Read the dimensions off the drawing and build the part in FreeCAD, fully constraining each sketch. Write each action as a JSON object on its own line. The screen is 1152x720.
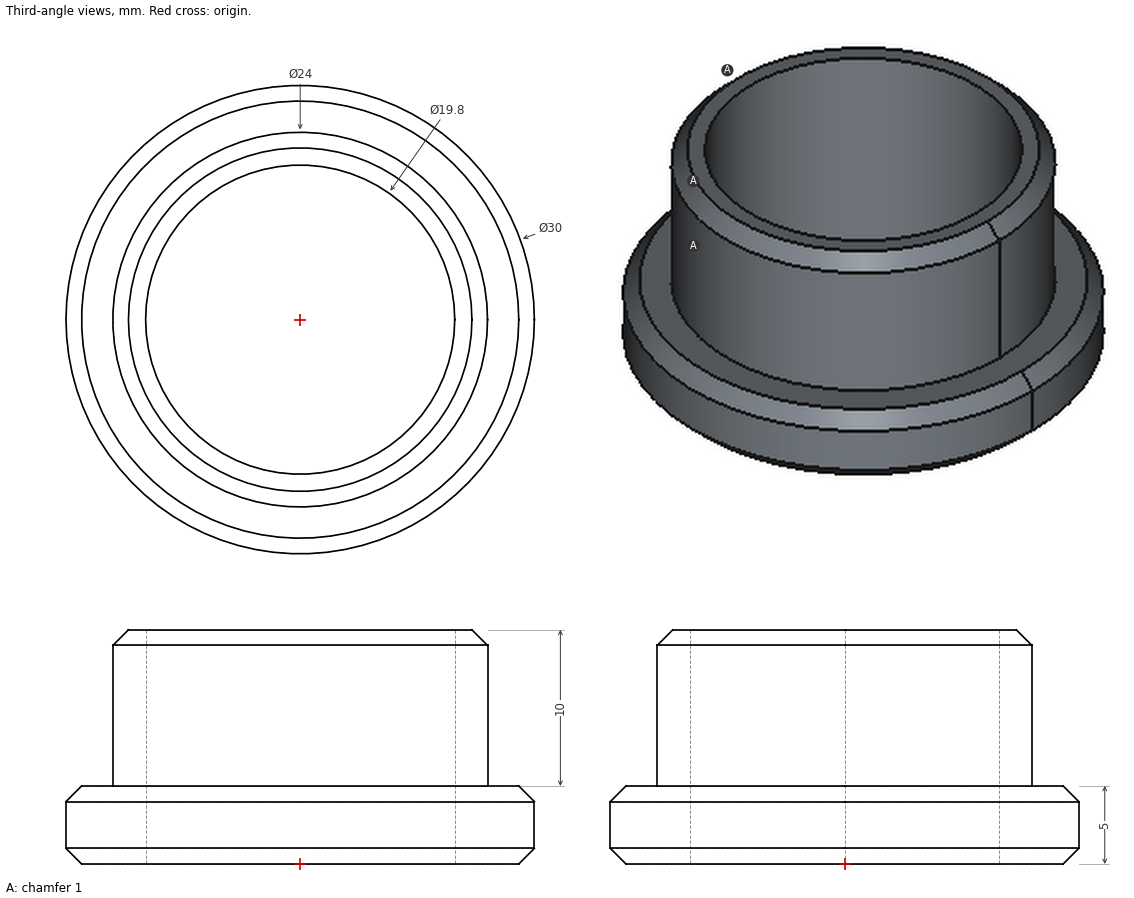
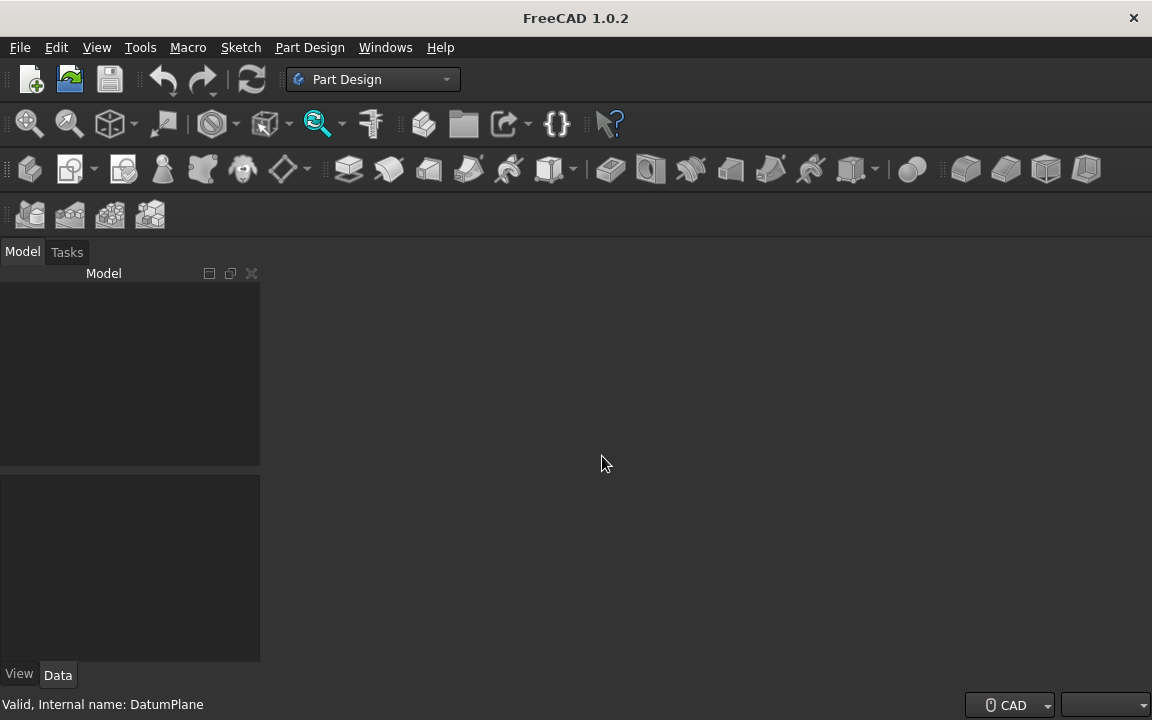
{"action": "left_click", "coordinate": [30, 80]}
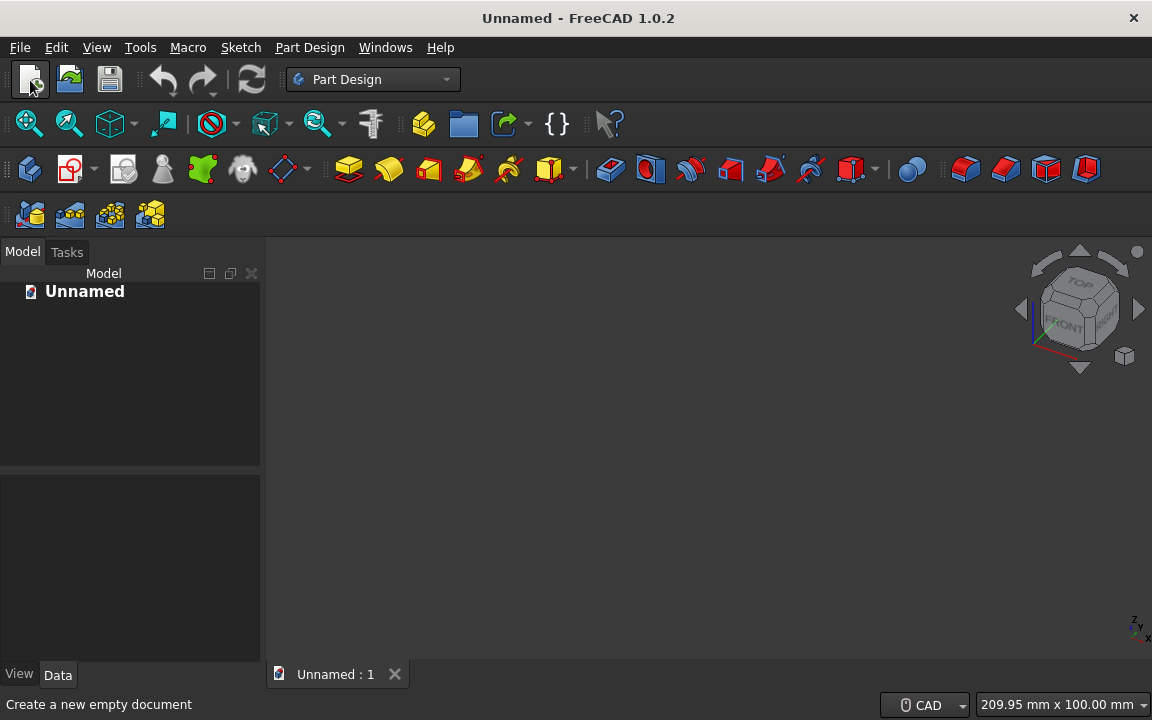
{"action": "left_click", "coordinate": [70, 170]}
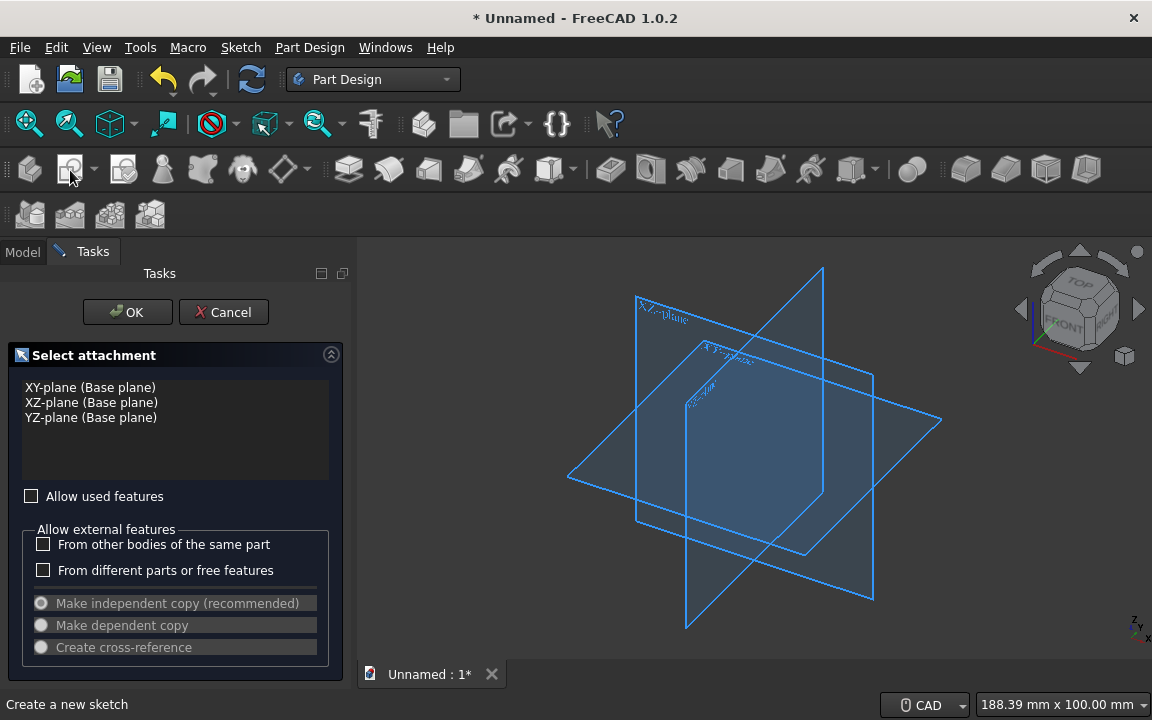
{"action": "left_click", "coordinate": [82, 388]}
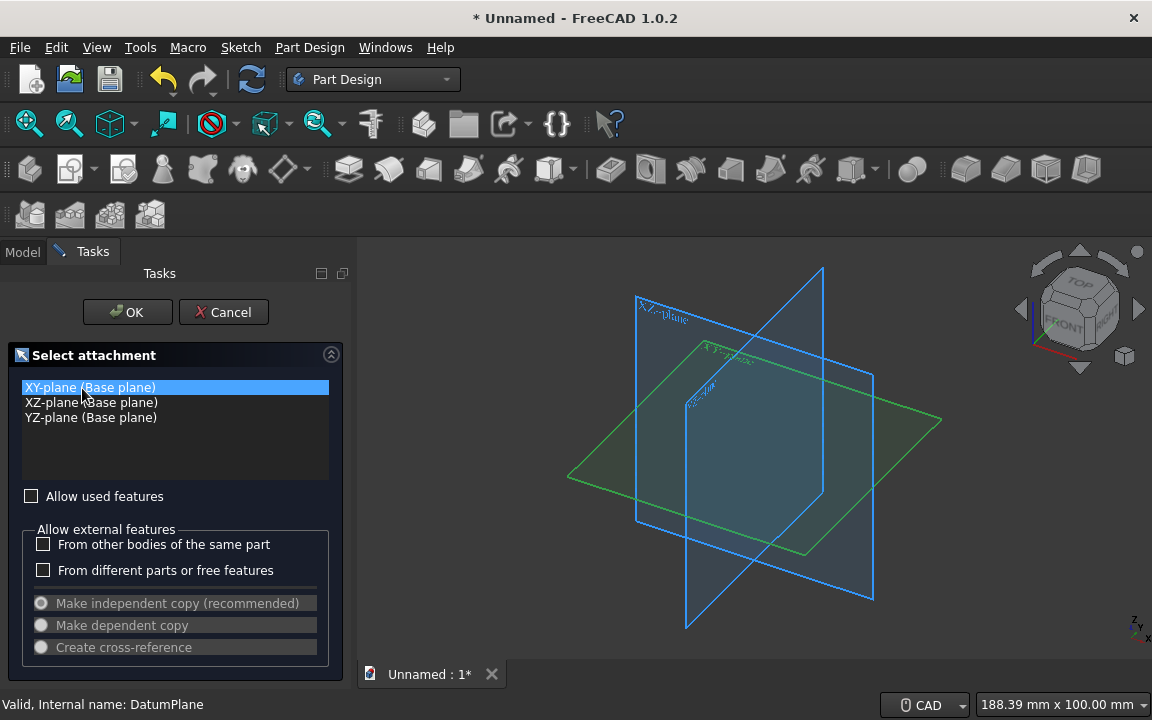
{"action": "left_click", "coordinate": [128, 312]}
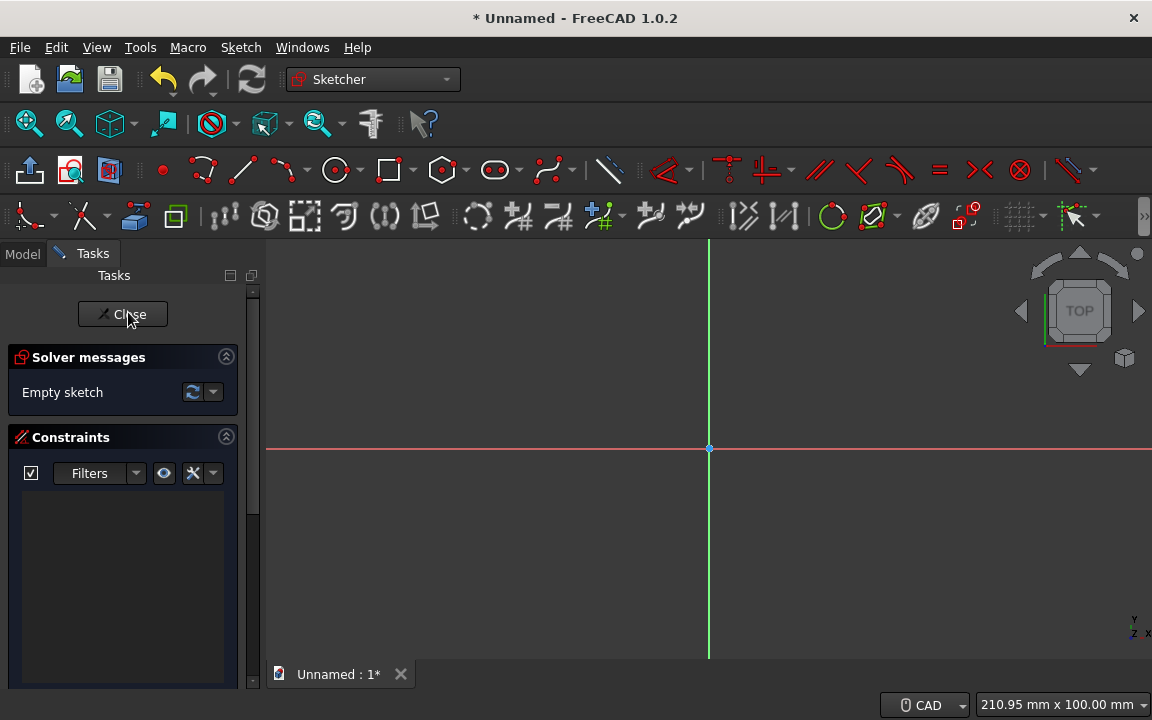
{"action": "scroll", "coordinate": [765, 449], "scroll_direction": "up", "scroll_amount": 4}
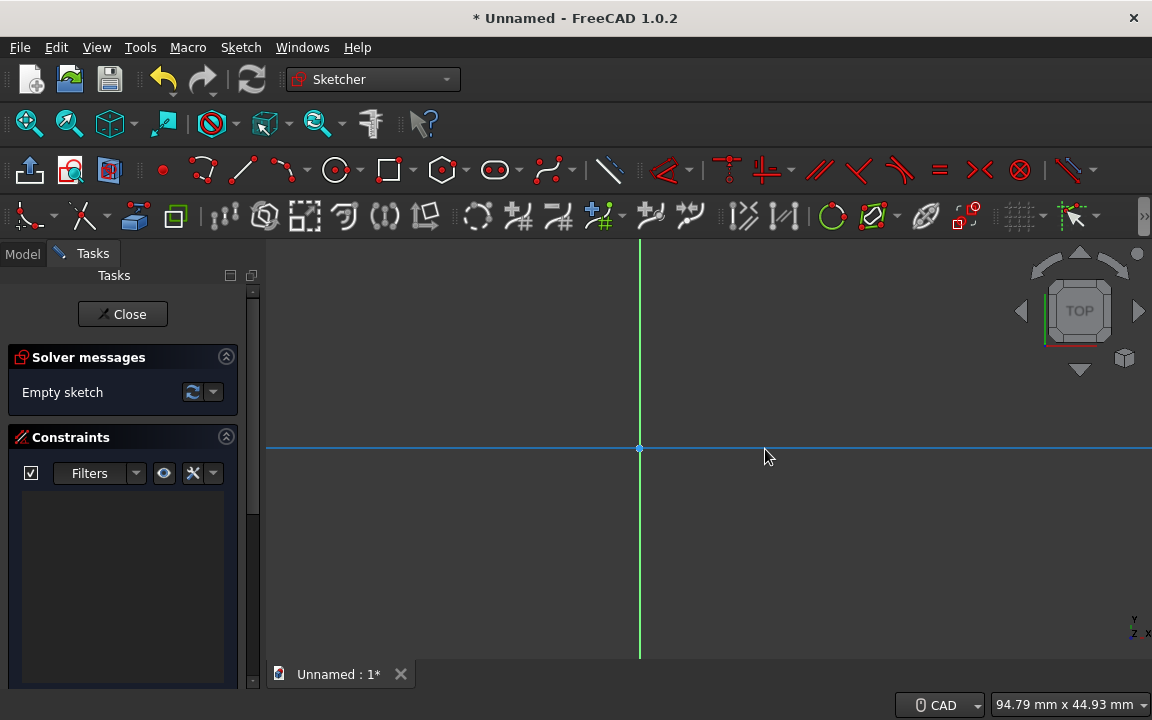
{"action": "key", "text": "g c"}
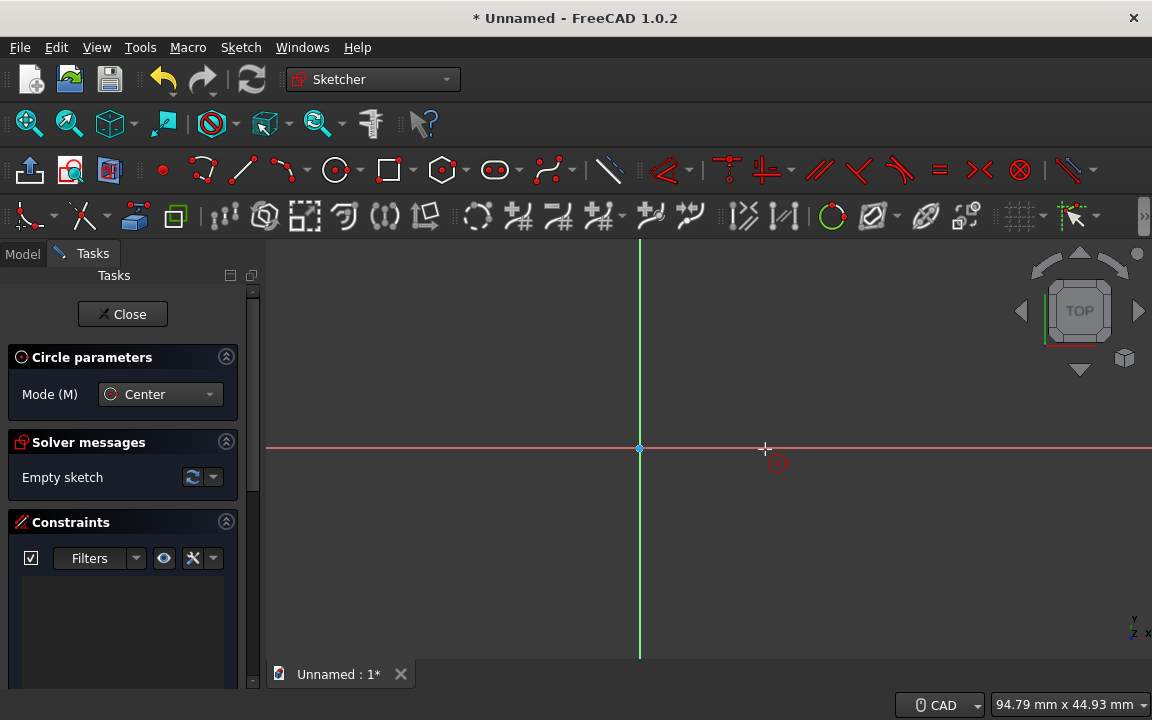
{"action": "left_click", "coordinate": [640, 448]}
{"action": "mouse_move", "coordinate": [739, 349]}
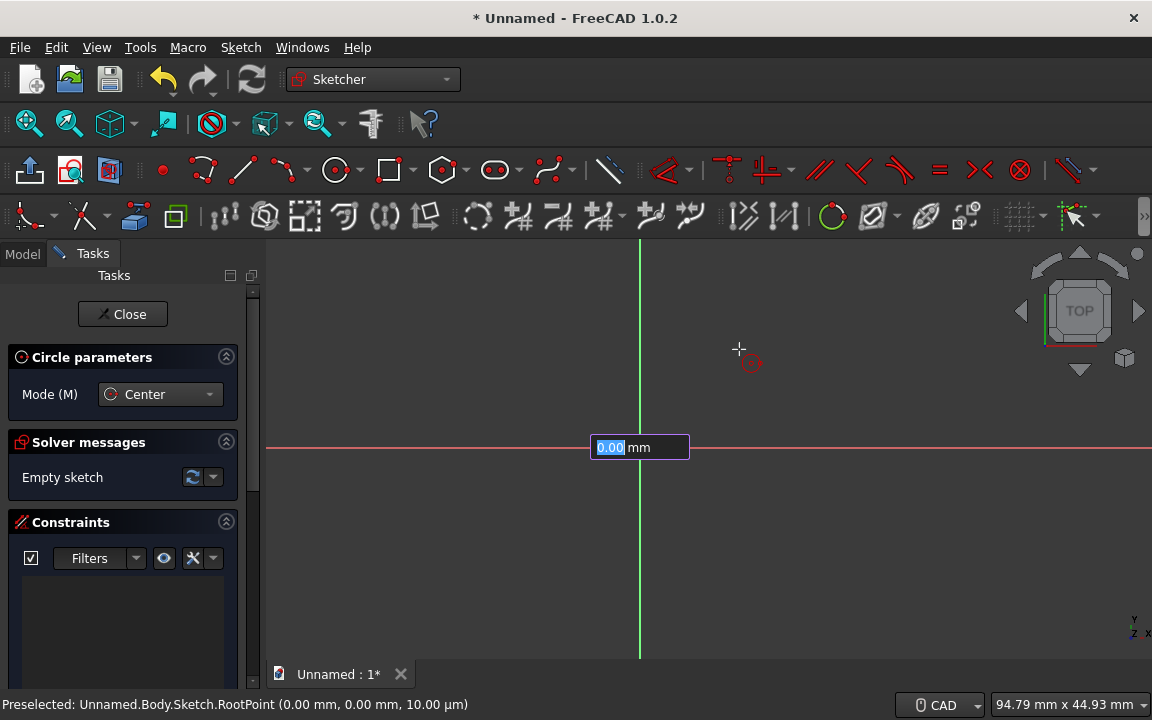
{"action": "type", "text": "30"}
{"action": "key", "text": "Return"}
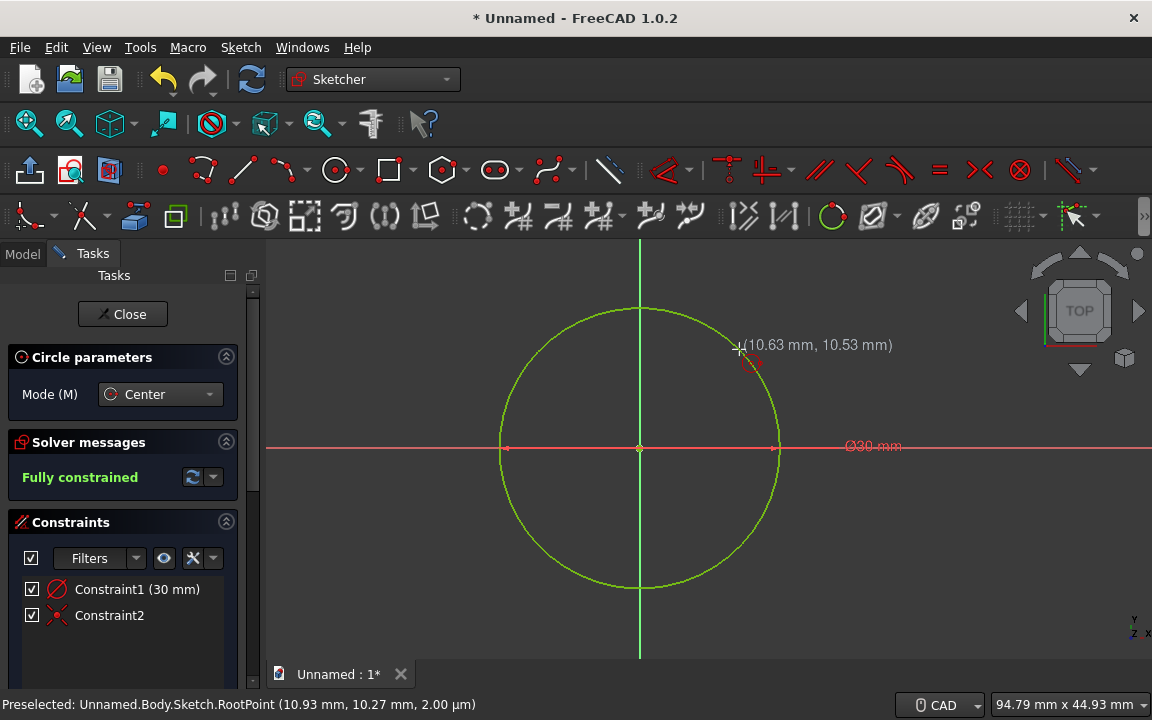
{"action": "left_click", "coordinate": [640, 448]}
{"action": "mouse_move", "coordinate": [705, 383]}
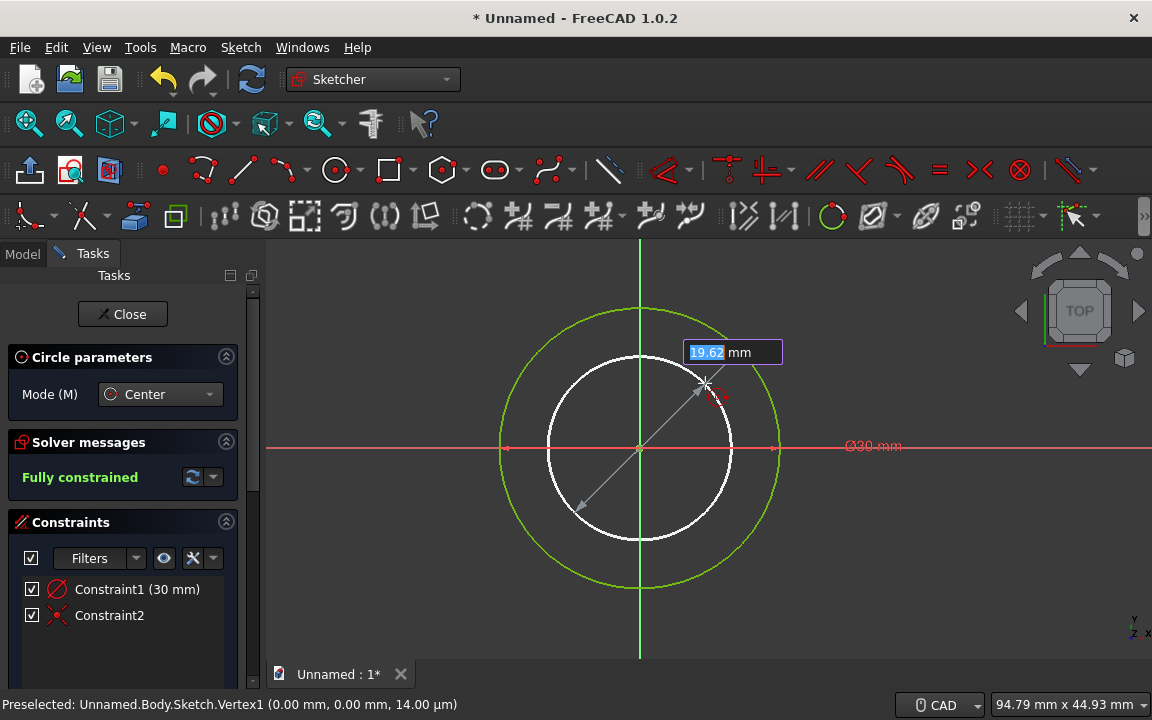
{"action": "type", "text": "19.8"}
{"action": "key", "text": "Return"}
{"action": "key", "text": "Escape"}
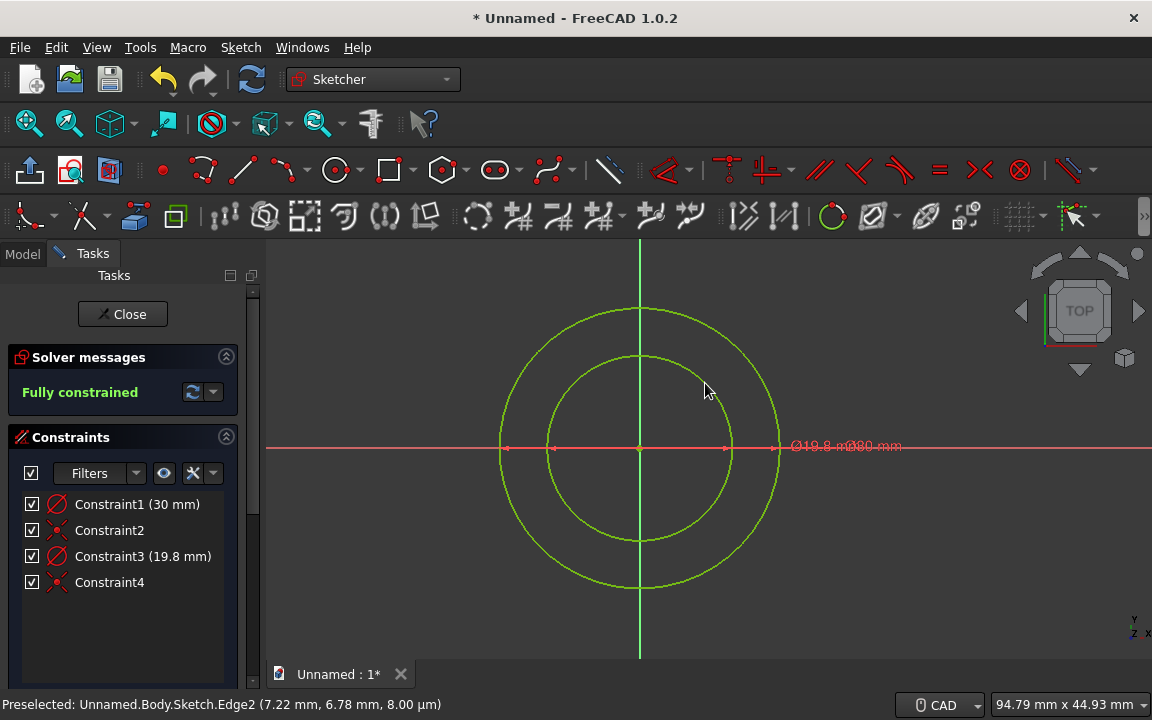
{"action": "left_click", "coordinate": [123, 314]}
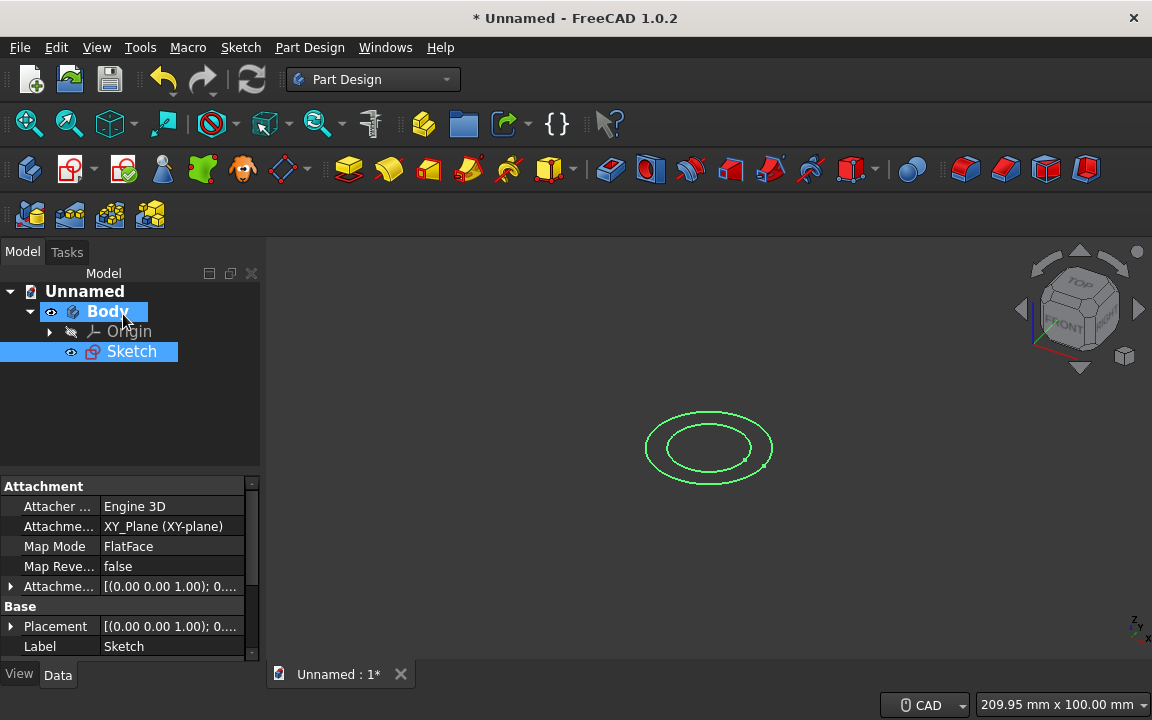
{"action": "left_click", "coordinate": [350, 170]}